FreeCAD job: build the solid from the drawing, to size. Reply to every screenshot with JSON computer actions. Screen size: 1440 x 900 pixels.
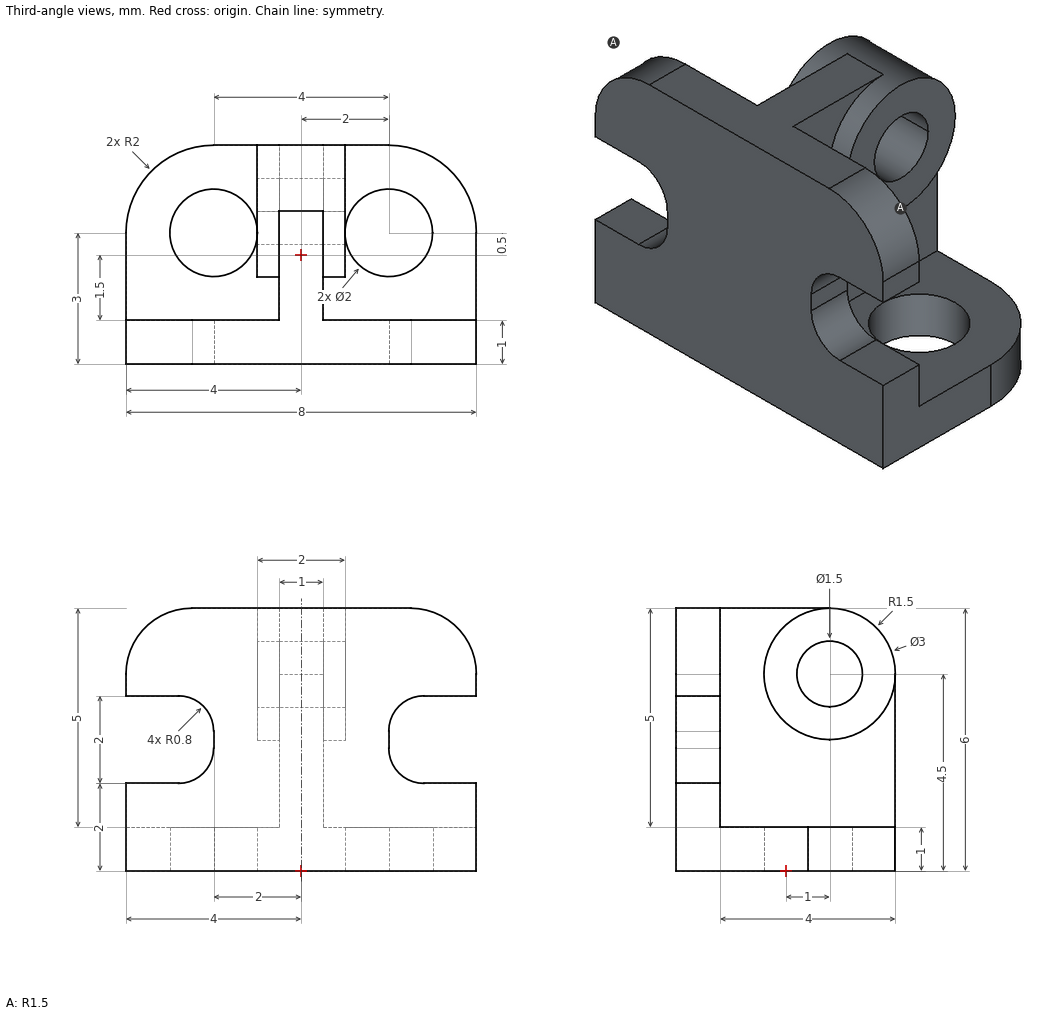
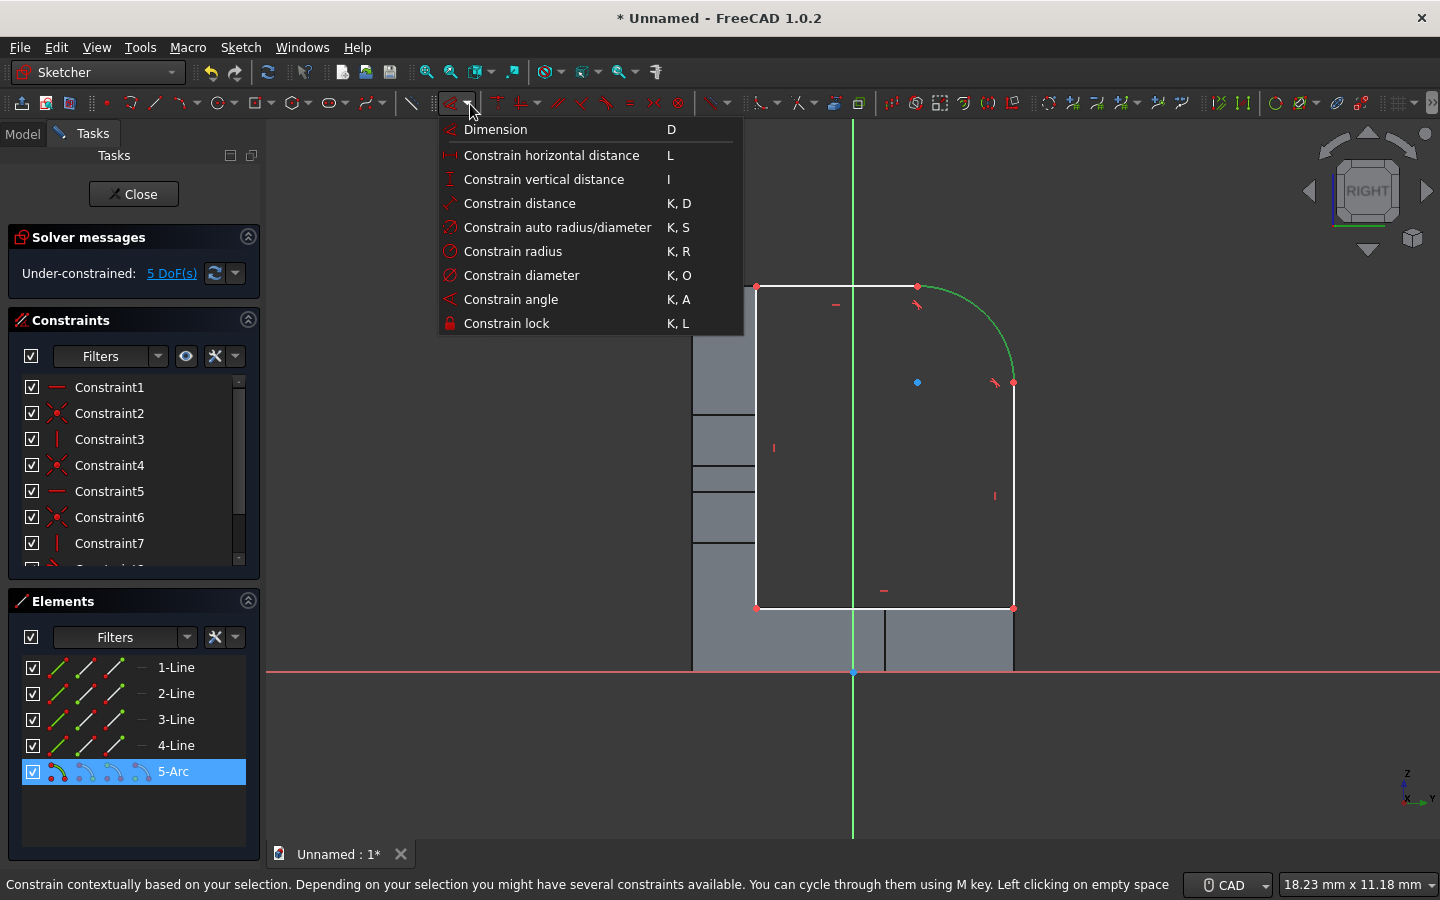
{"action": "left_click", "coordinate": [591, 251]}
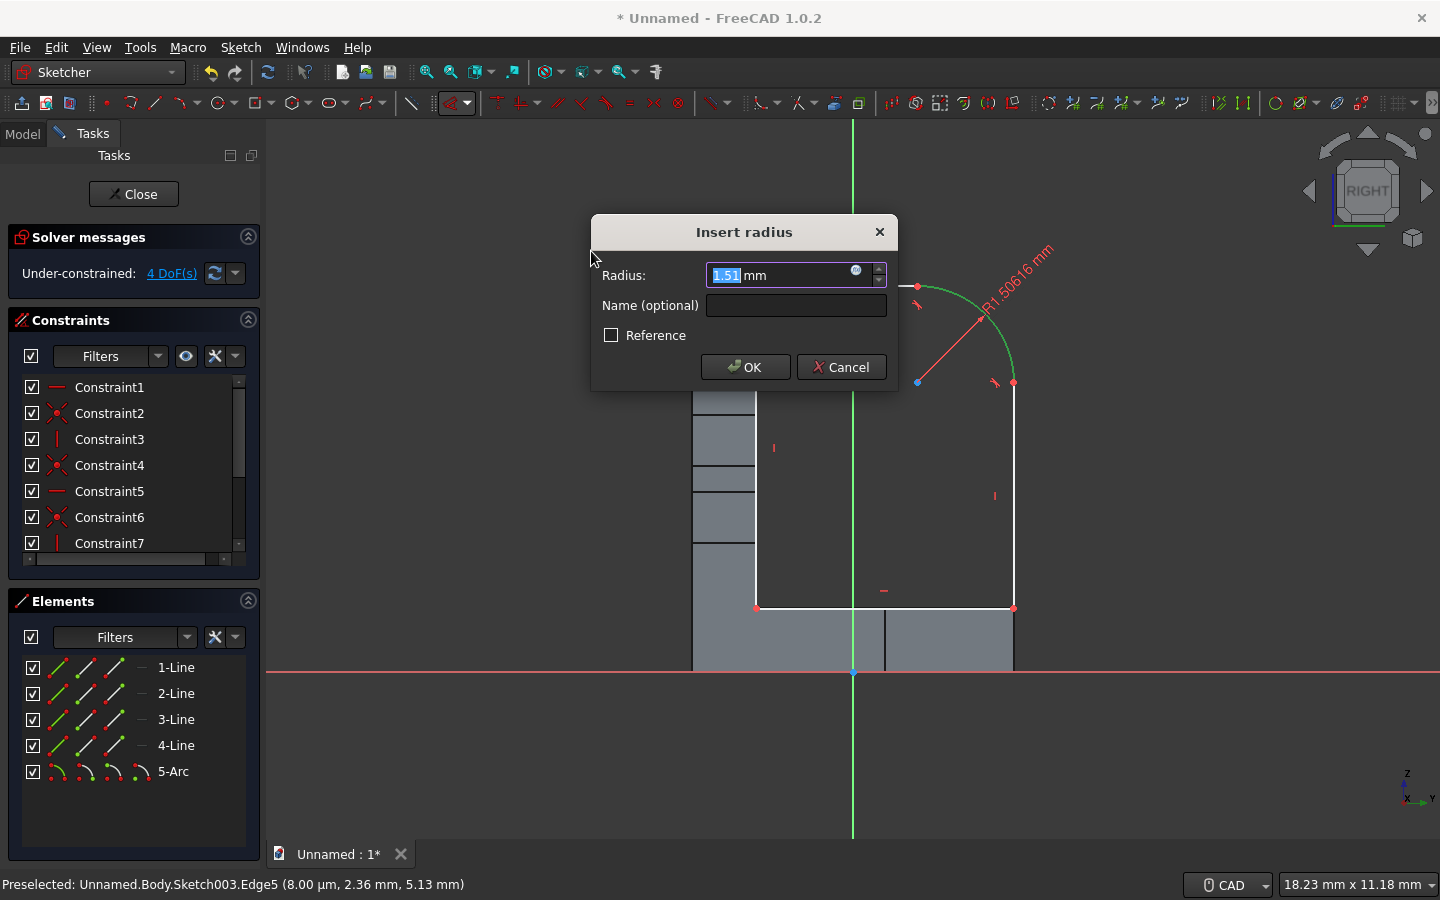
{"action": "type", "text": "1.5"}
{"action": "key", "text": "Return"}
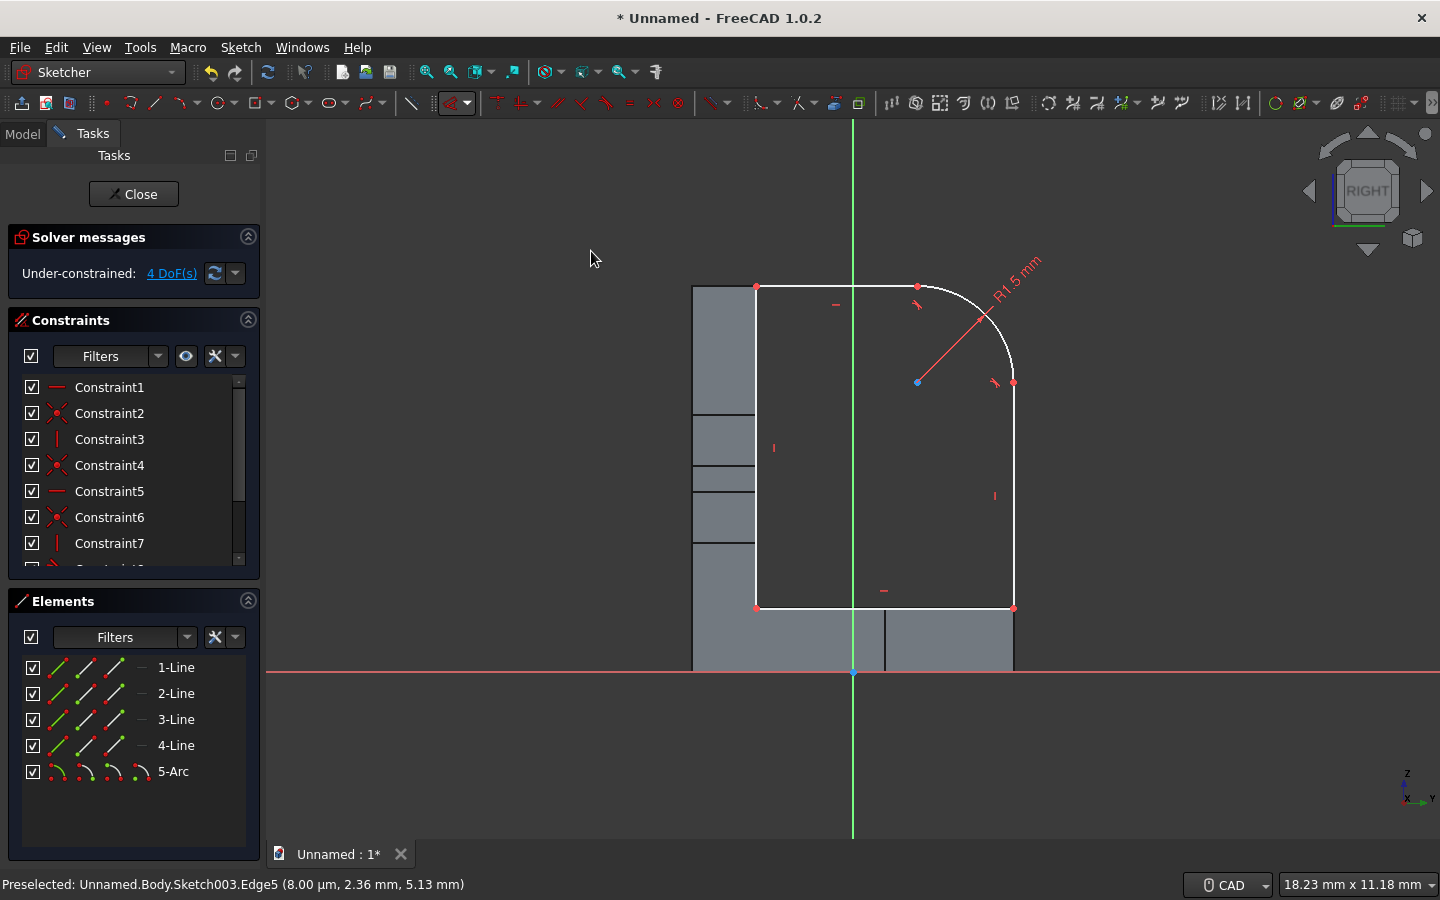
{"action": "left_click", "coordinate": [756, 383]}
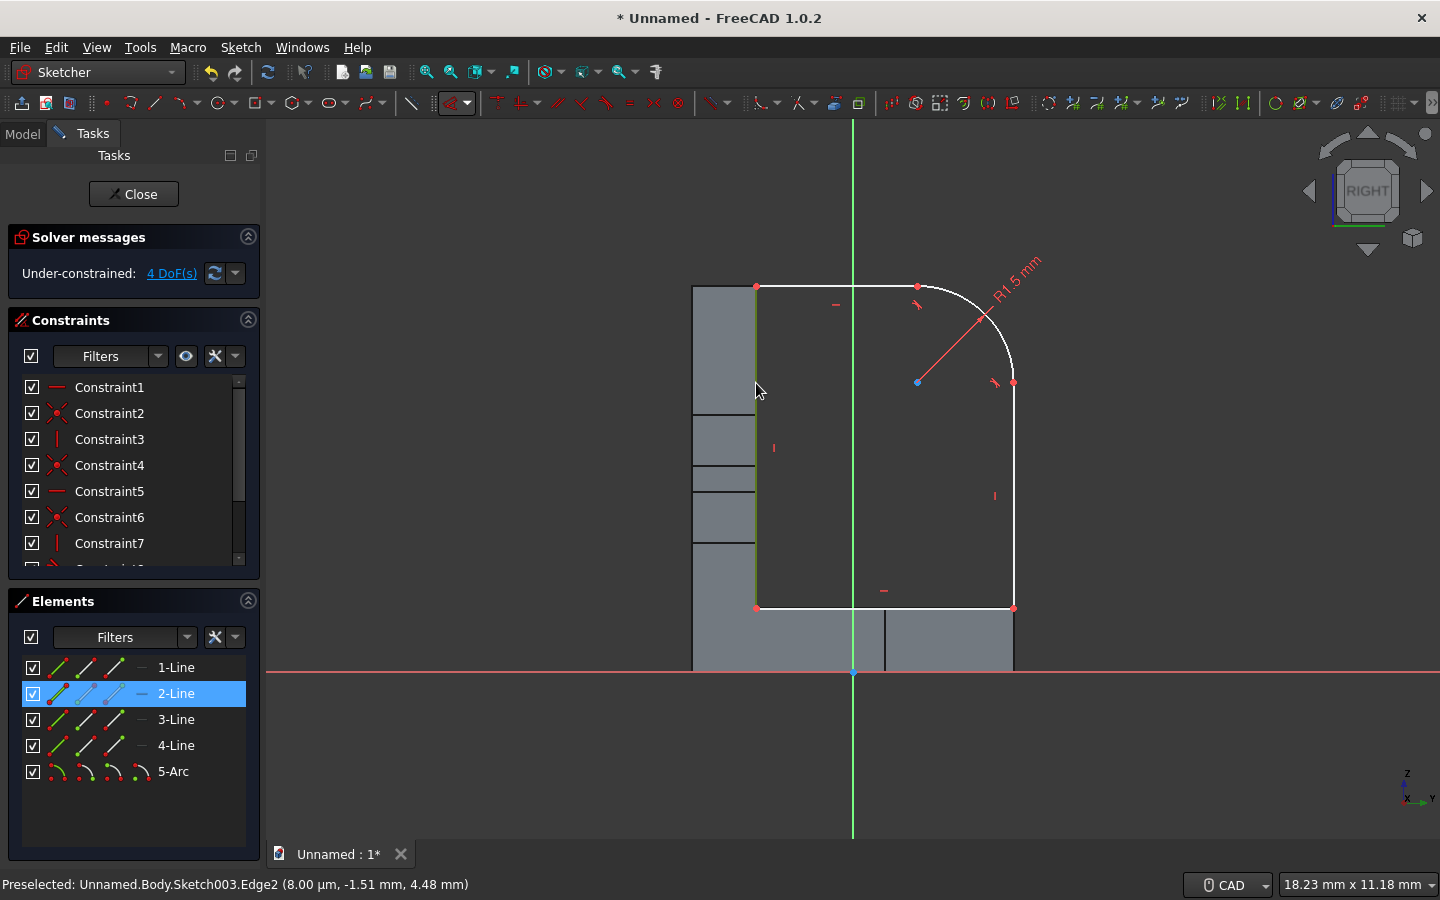
{"action": "left_click", "coordinate": [470, 104]}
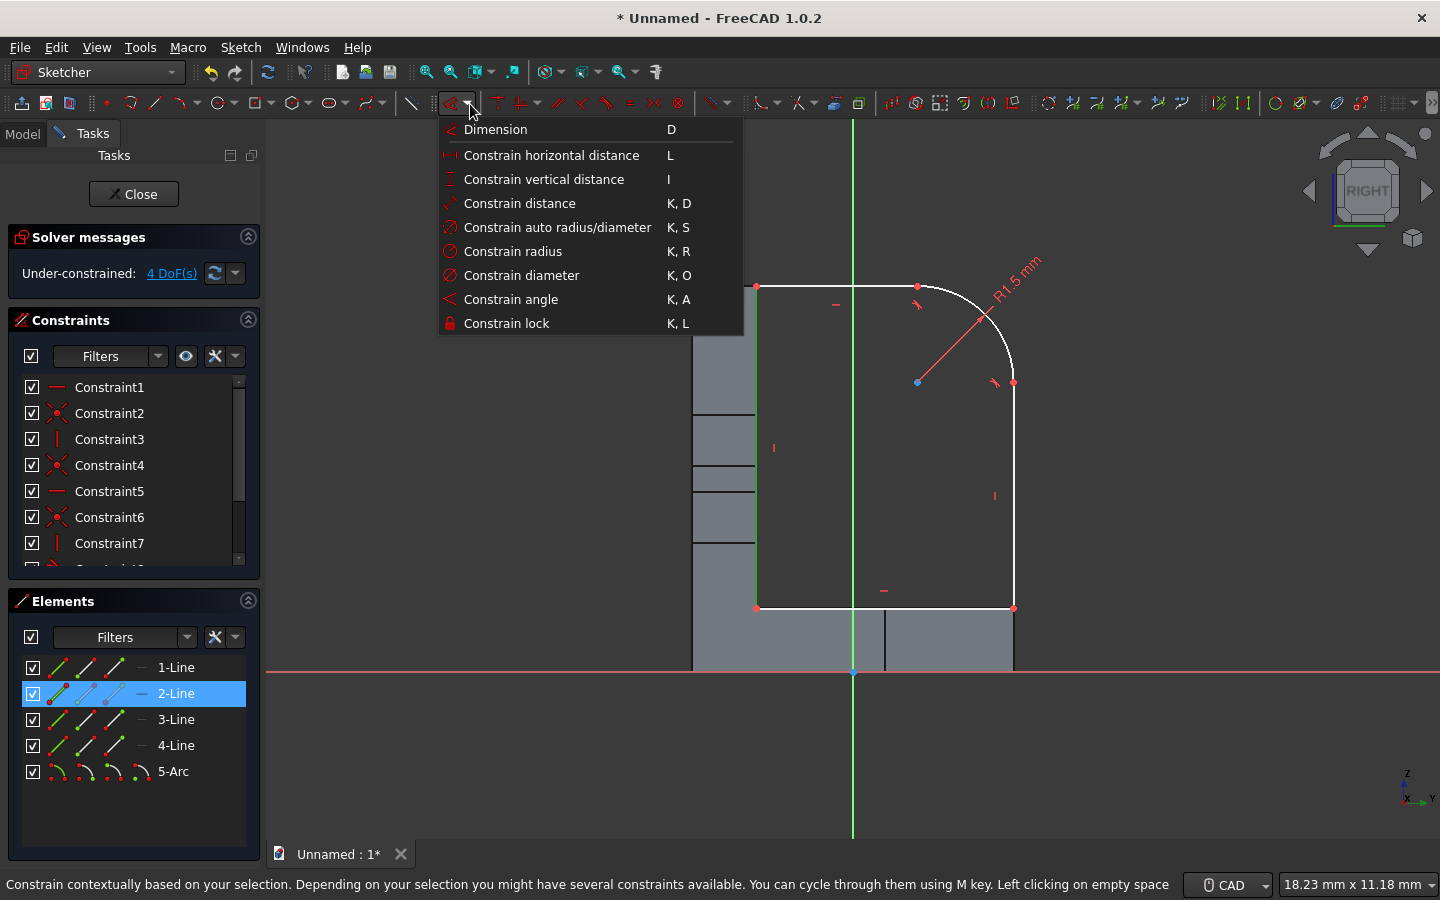
{"action": "left_click", "coordinate": [591, 179]}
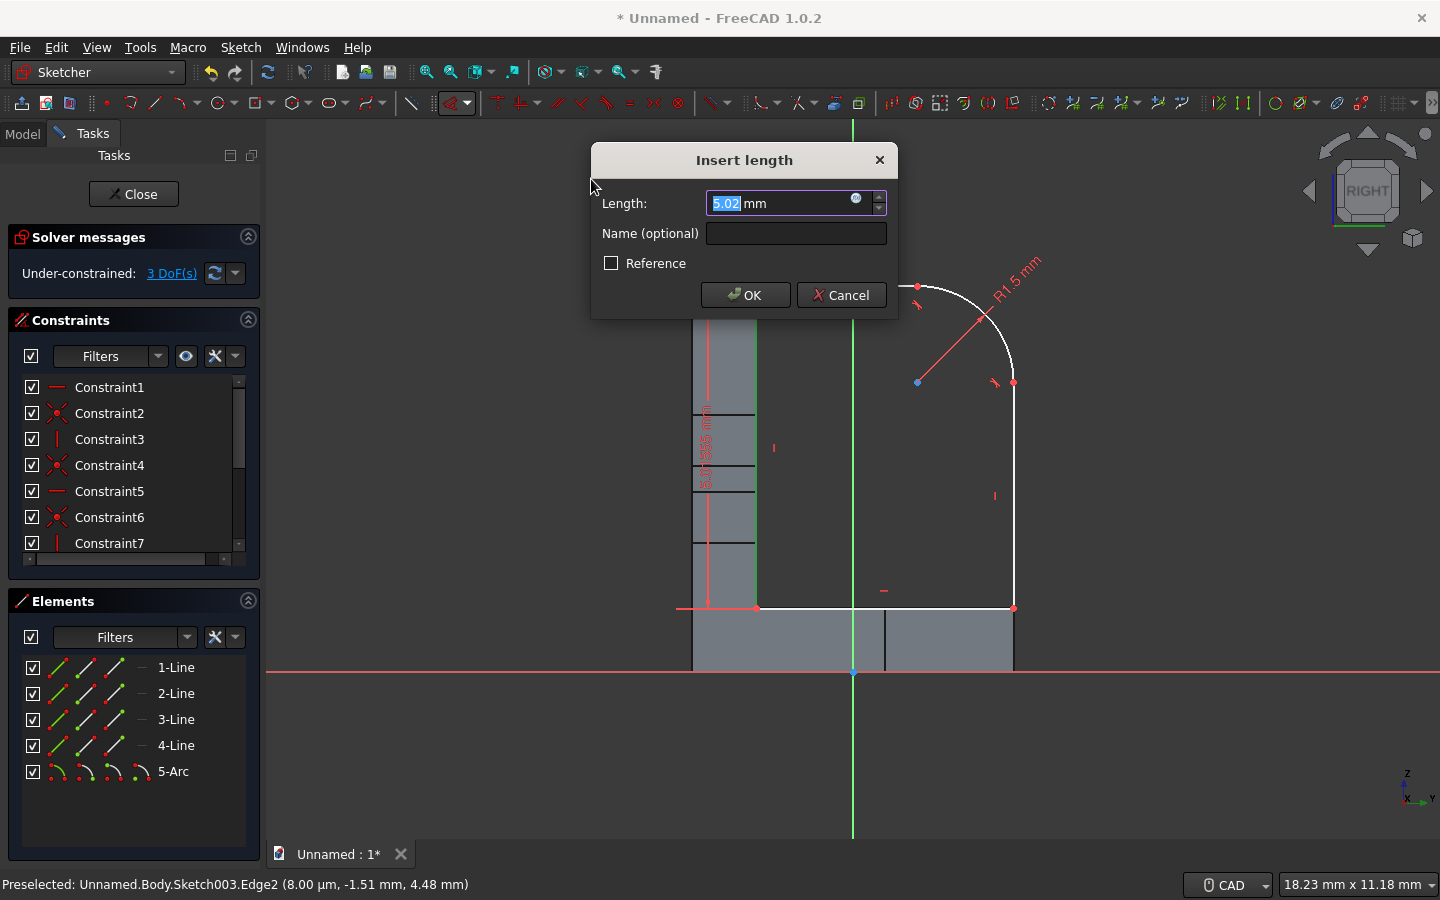
{"action": "type", "text": "5"}
{"action": "key", "text": "Return"}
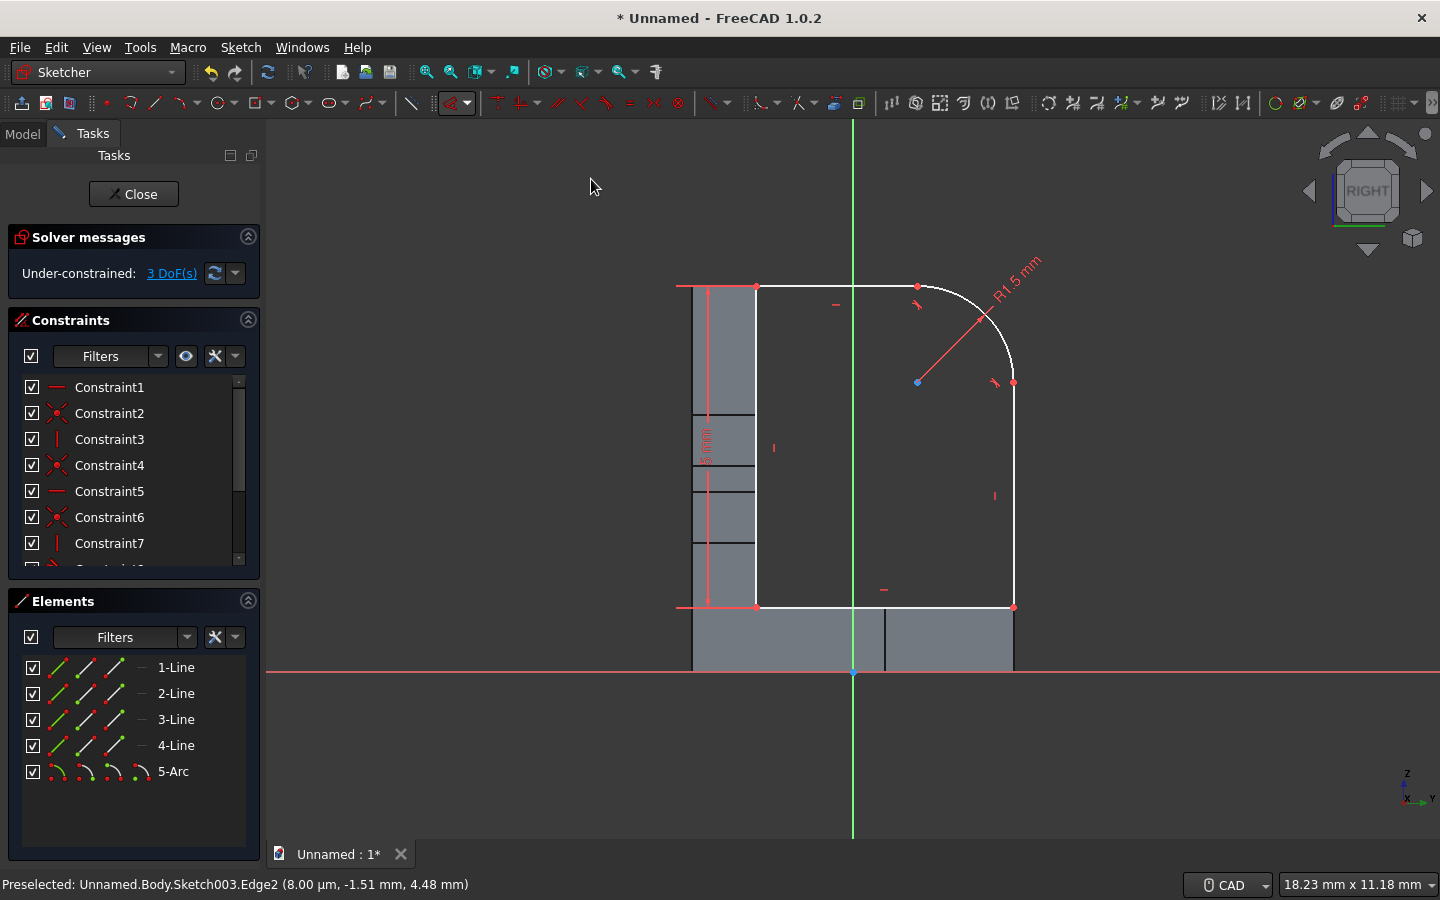
{"action": "left_click", "coordinate": [833, 608]}